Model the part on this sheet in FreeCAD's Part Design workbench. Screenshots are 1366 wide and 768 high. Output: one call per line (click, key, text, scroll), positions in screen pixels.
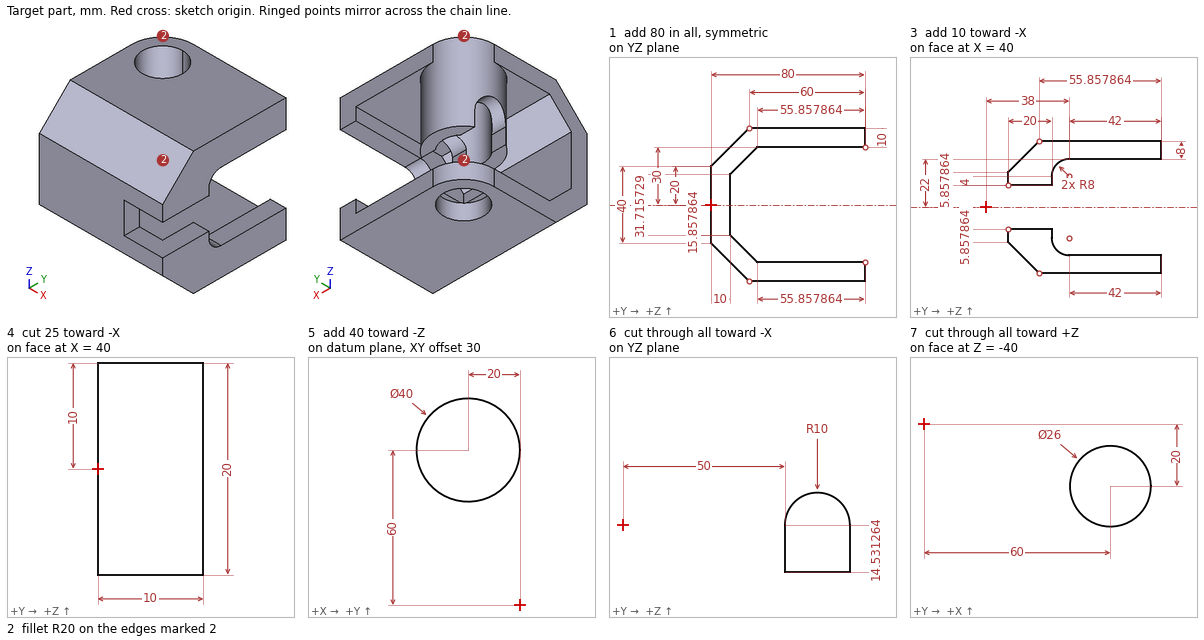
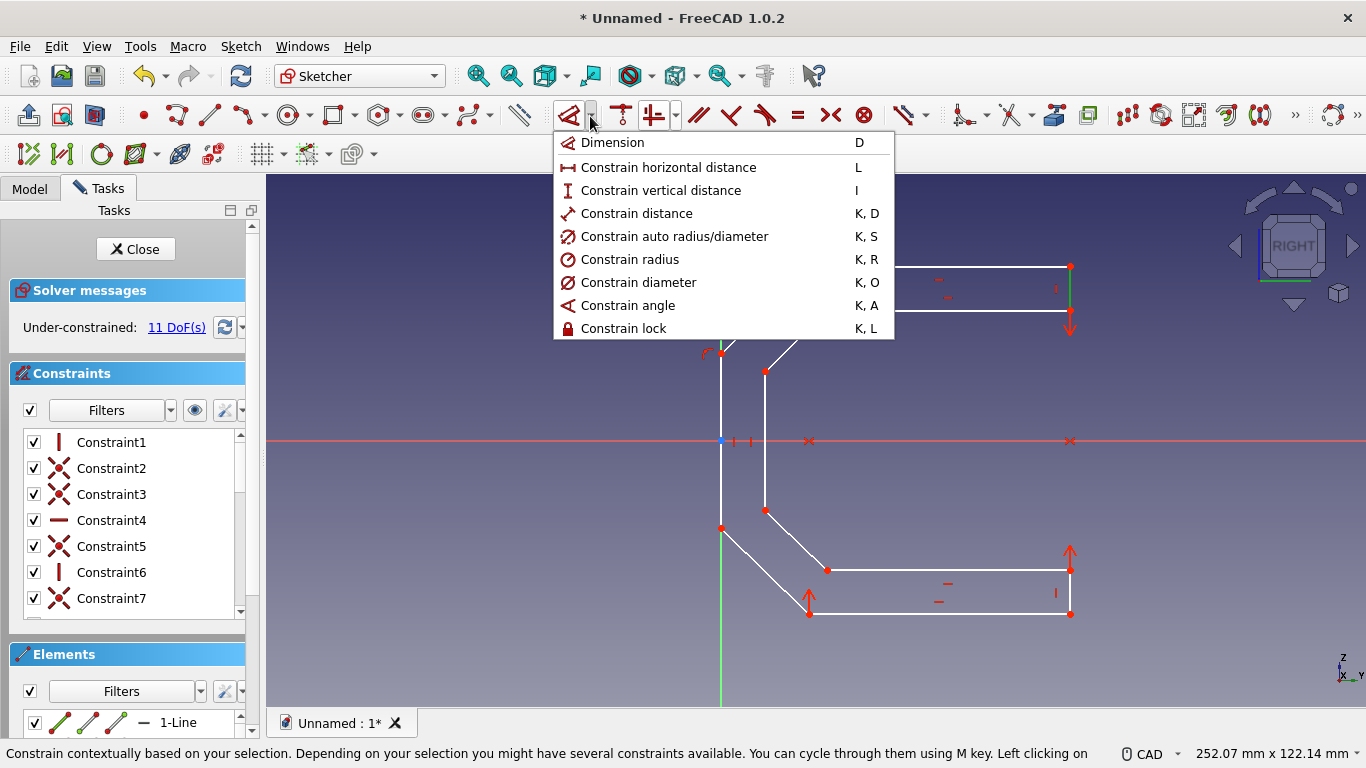
click(724, 190)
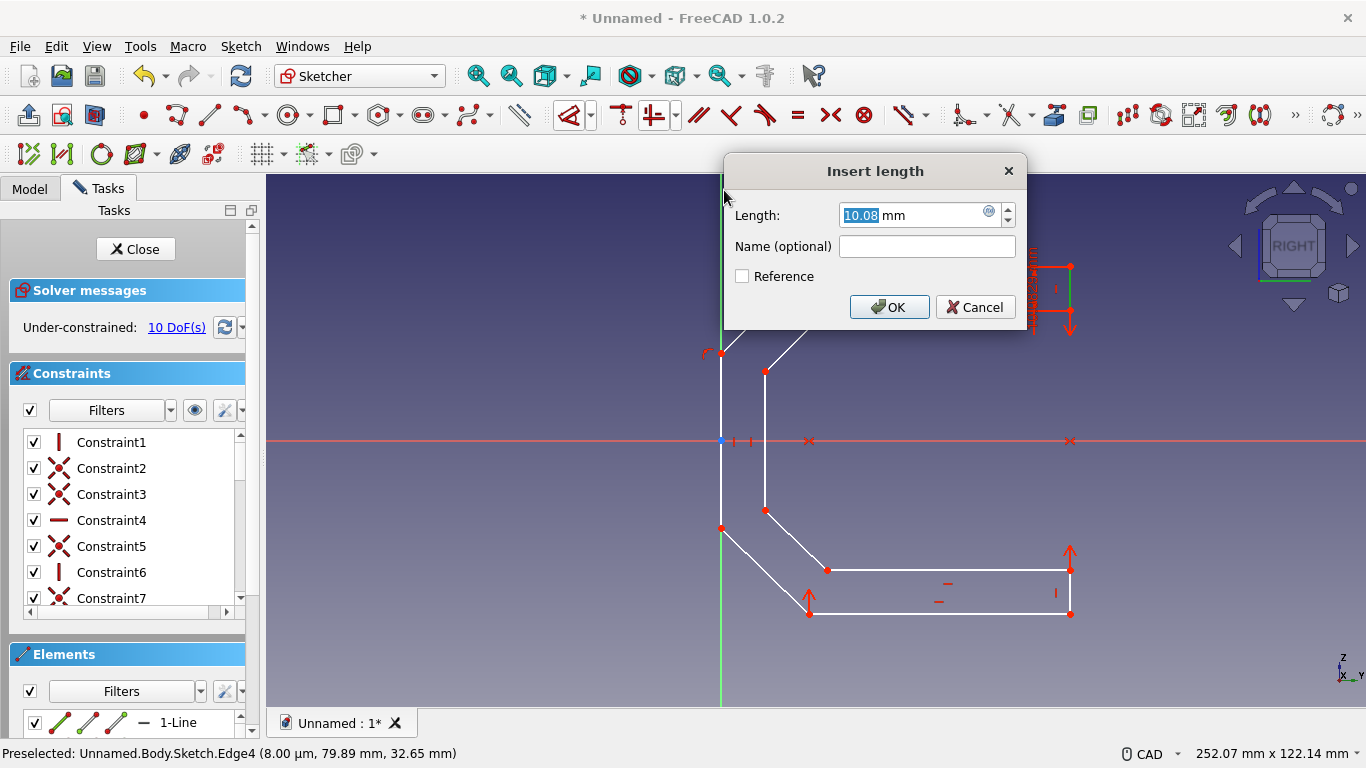
text(10)
key(Return)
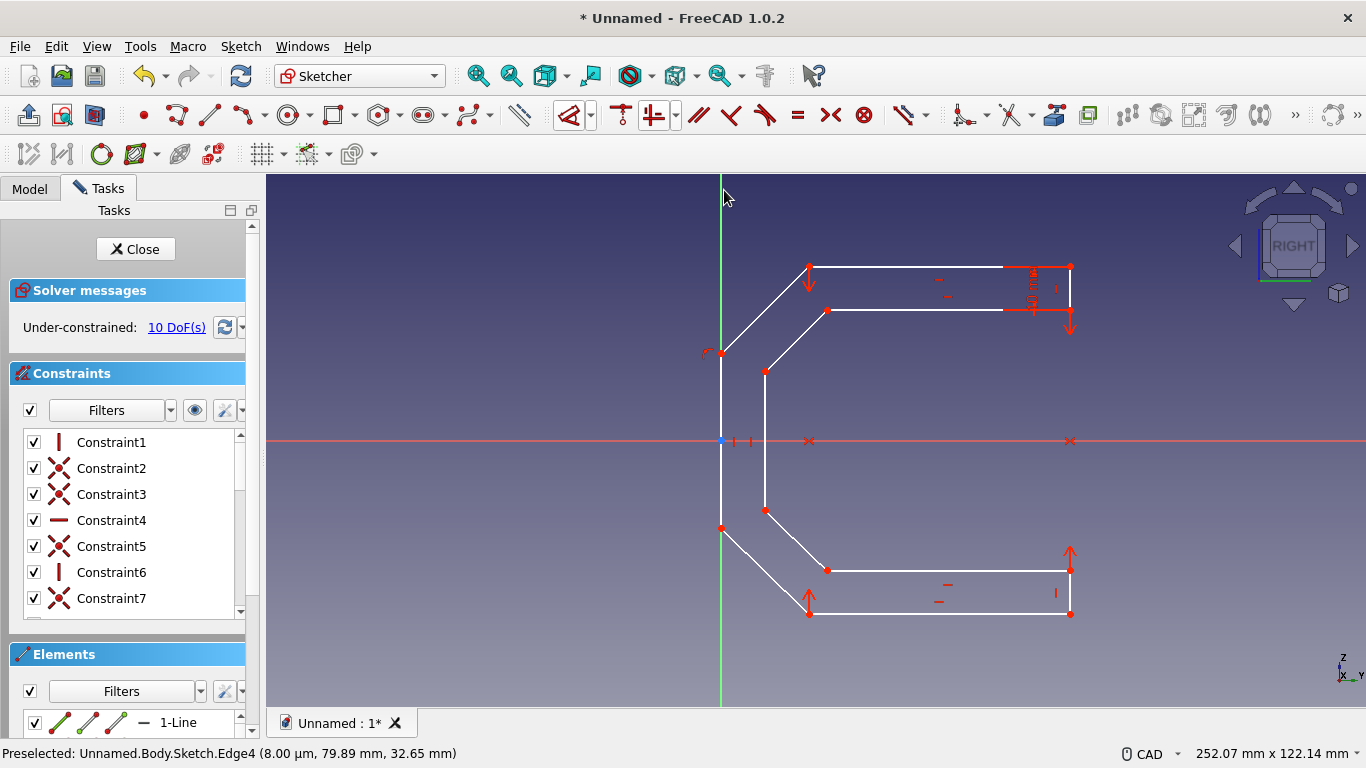
click(992, 267)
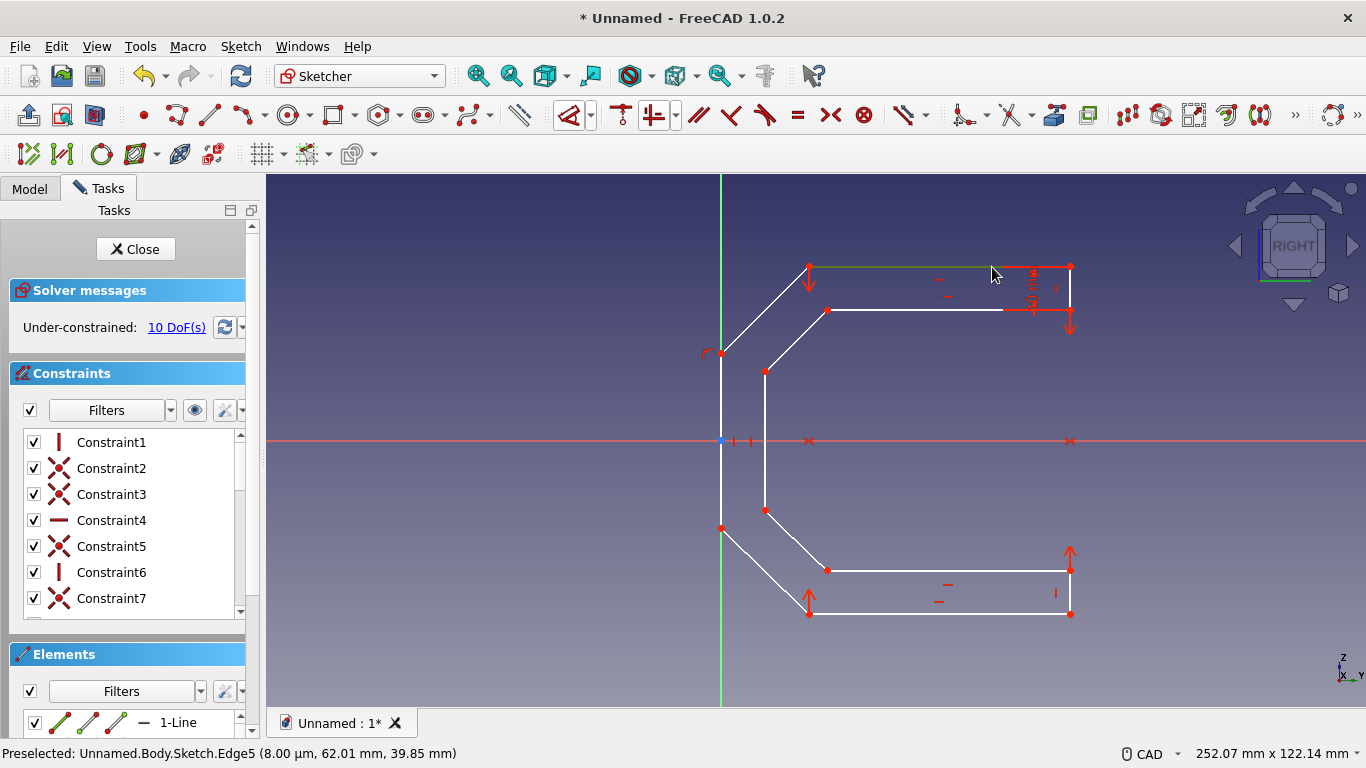
click(590, 116)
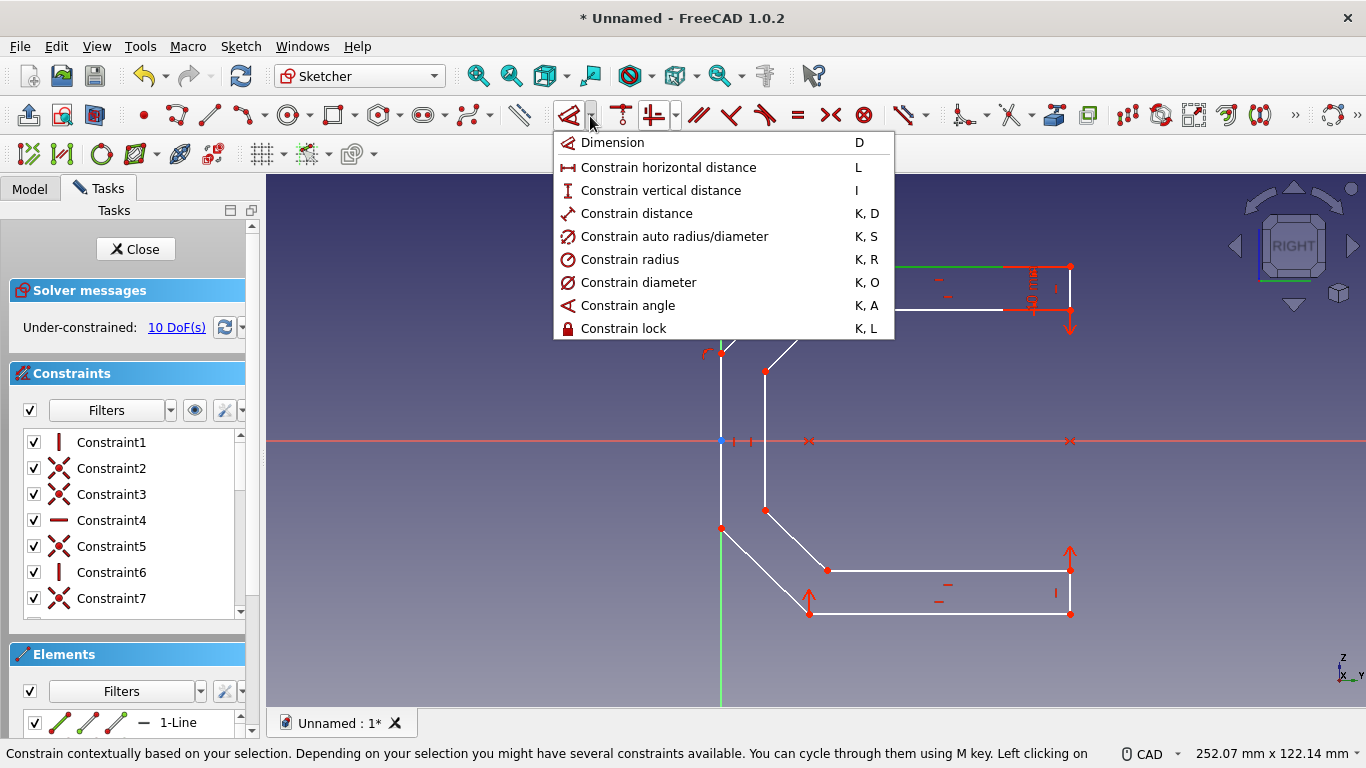
click(724, 168)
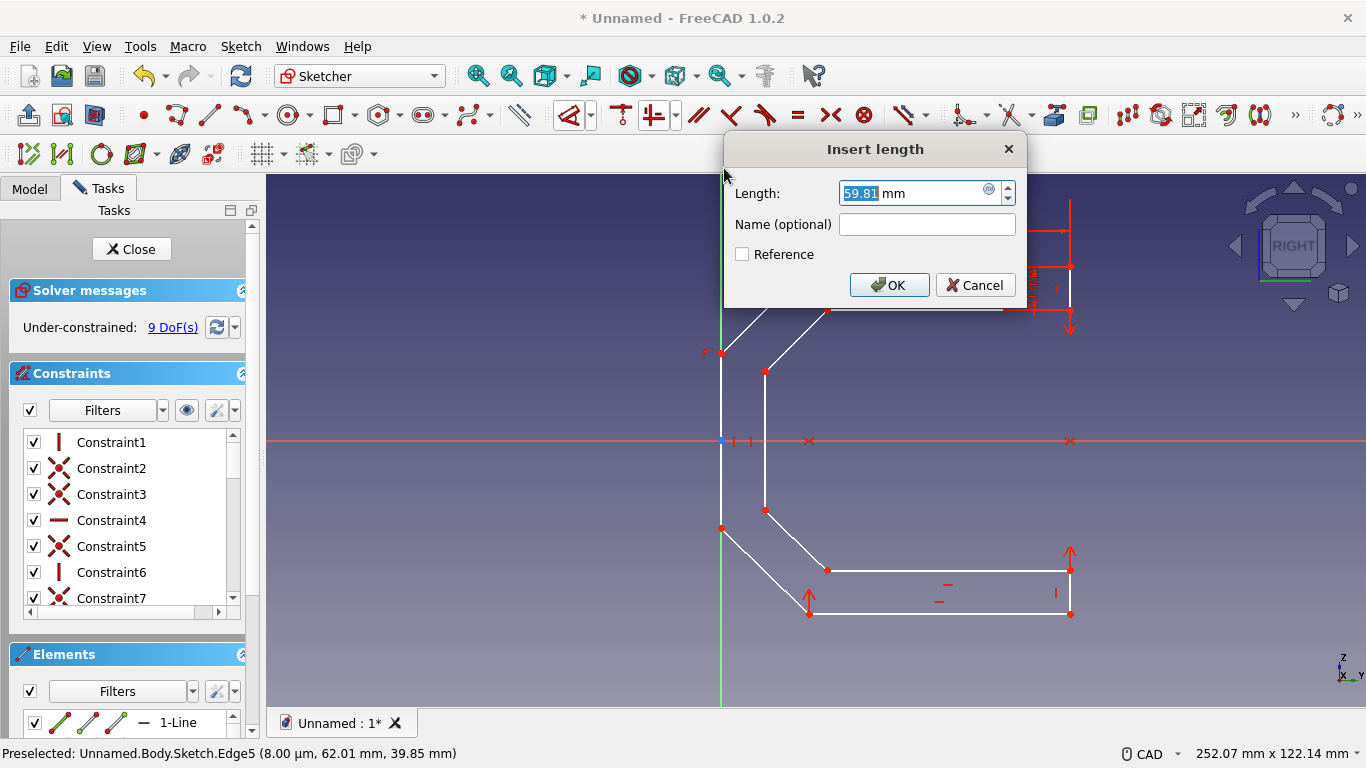
text(60)
key(Return)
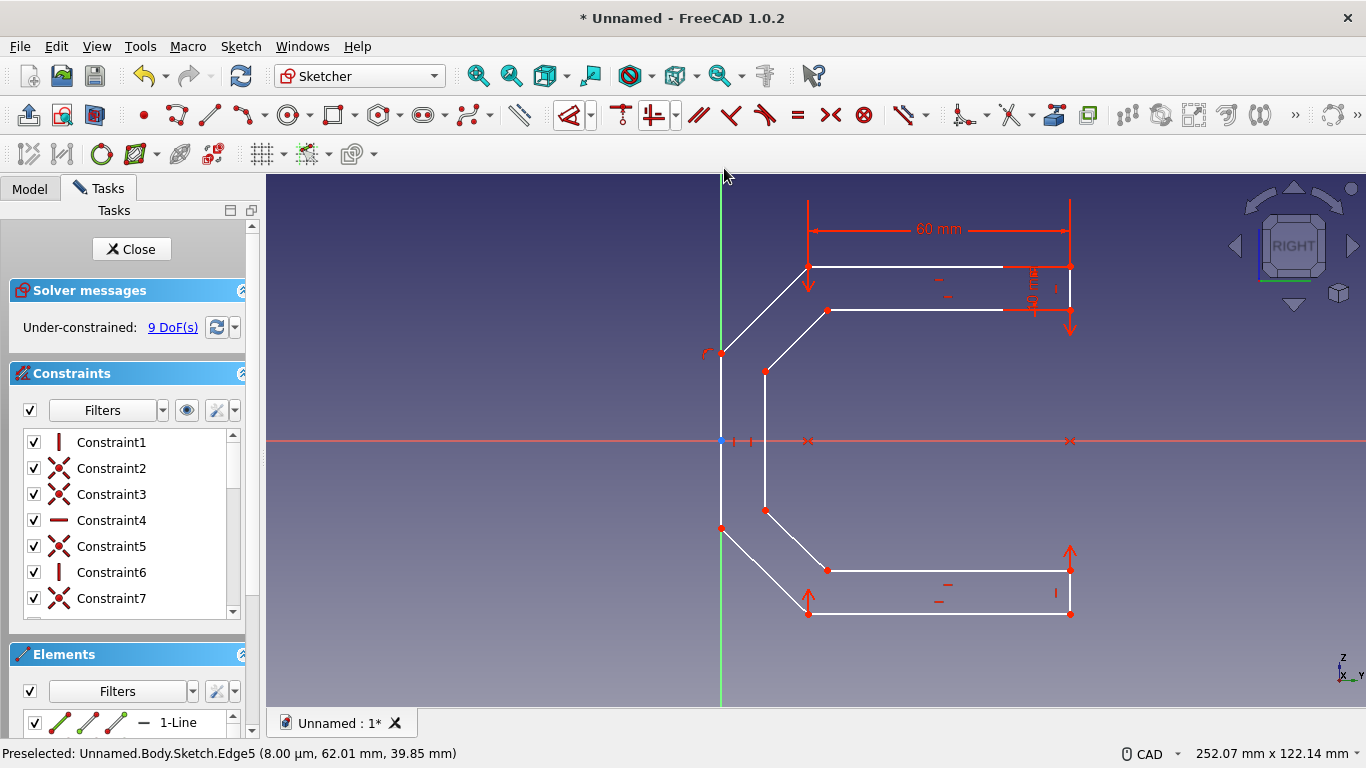
click(721, 407)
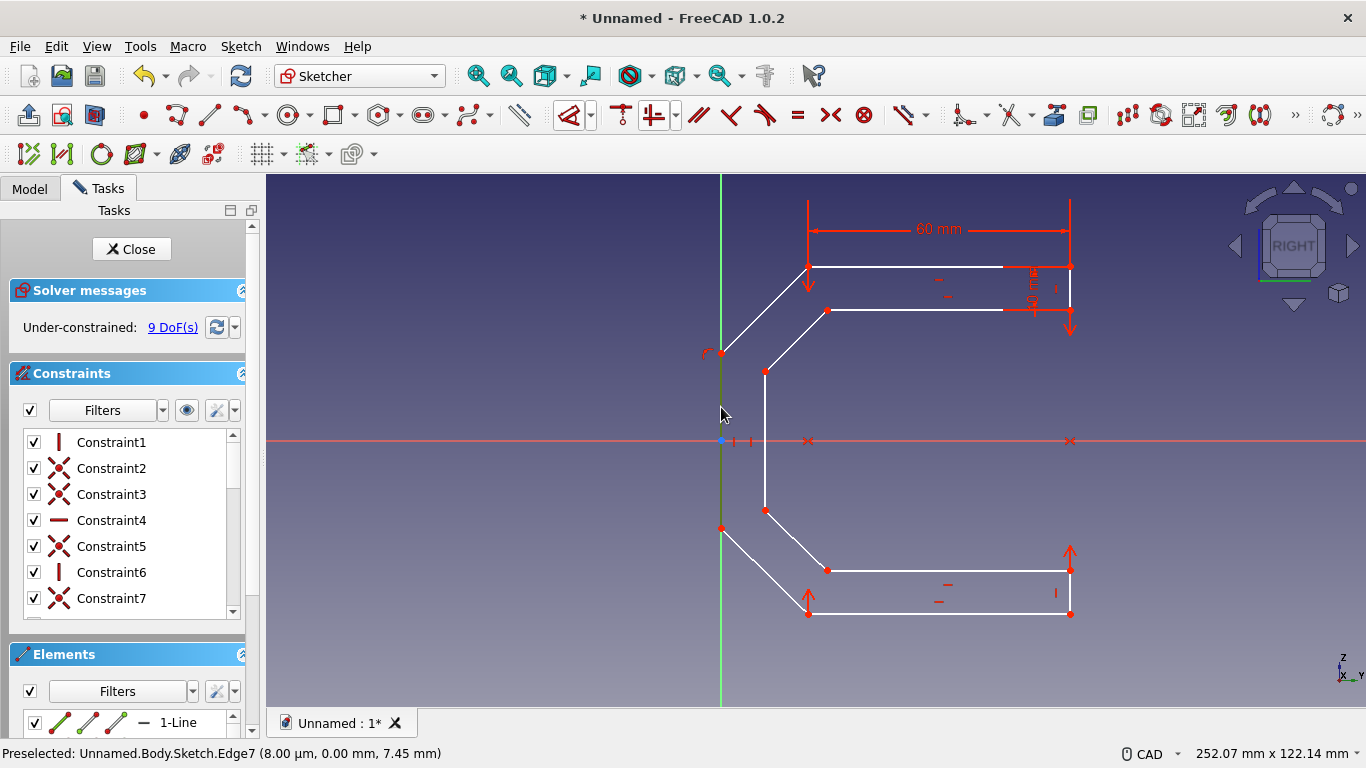
click(590, 116)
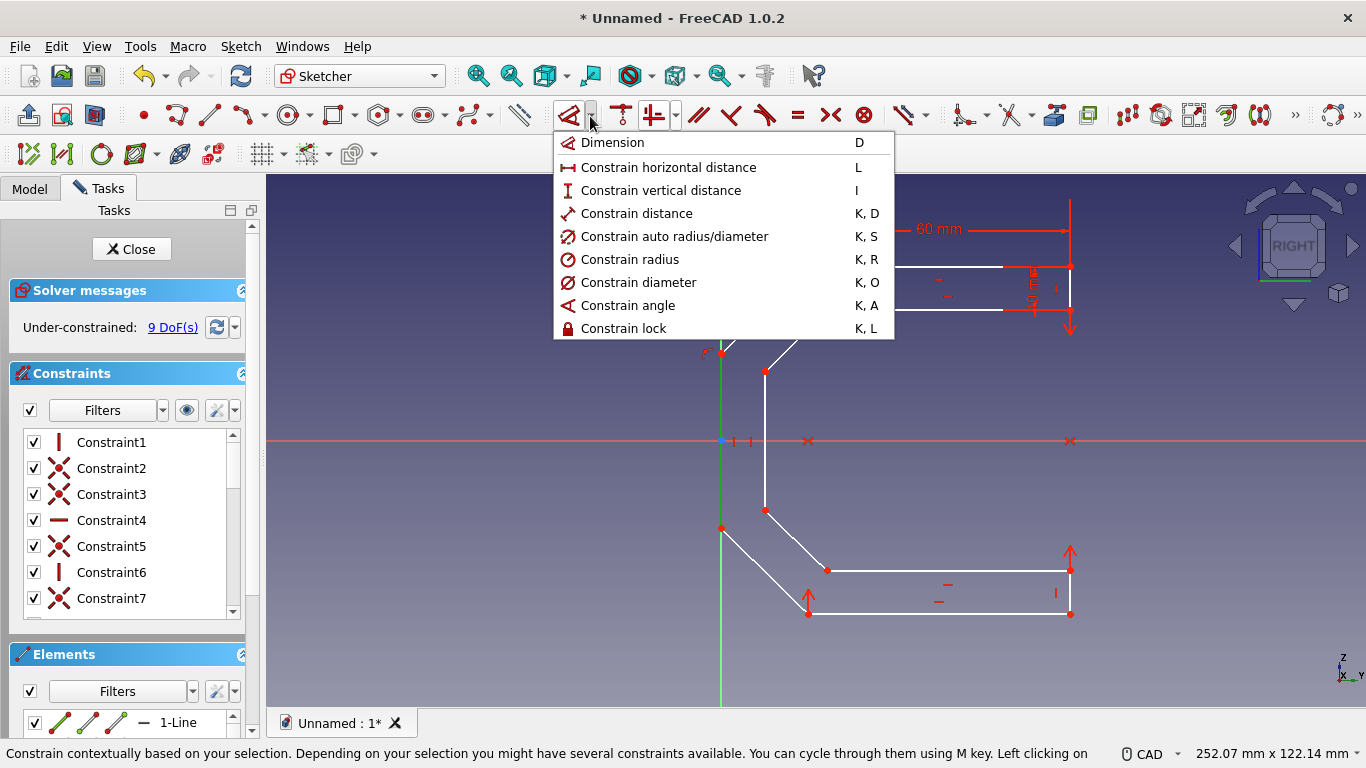
click(724, 190)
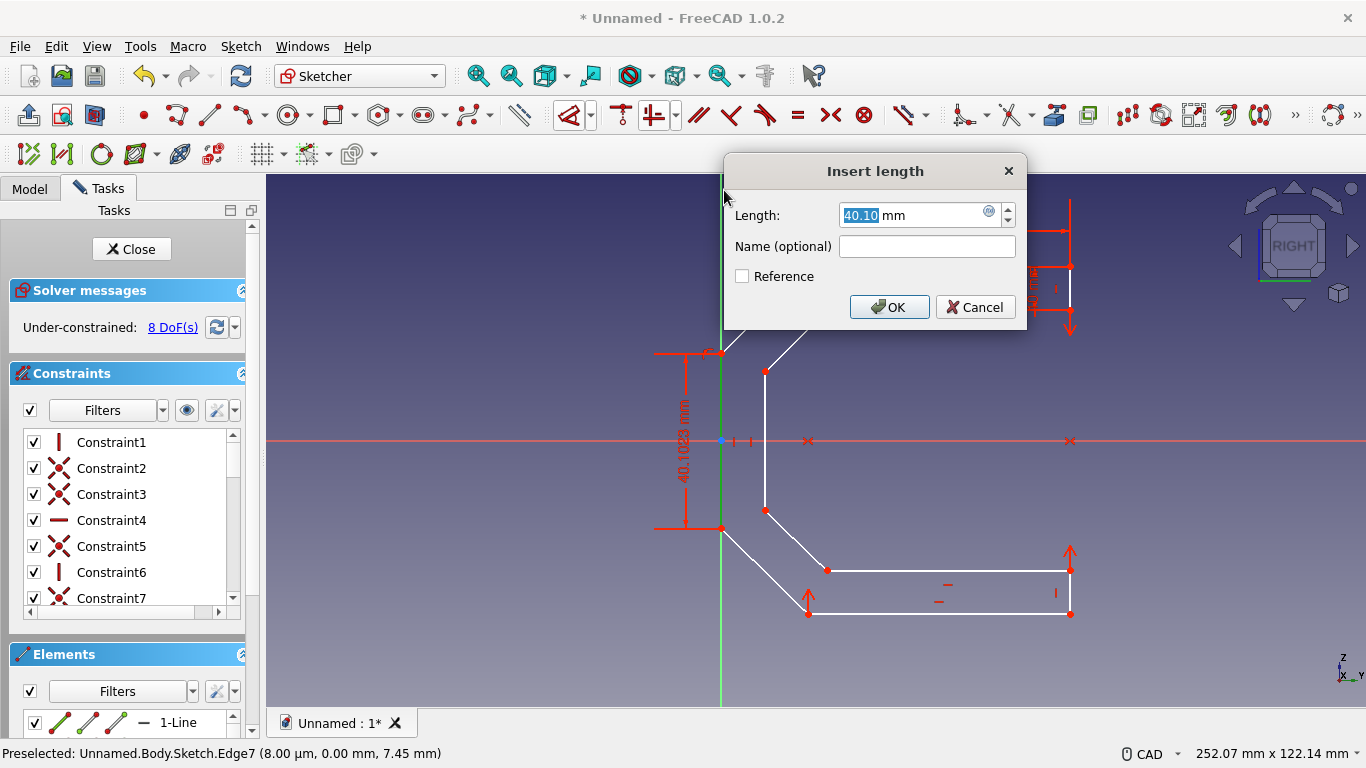
text(40)
key(Return)